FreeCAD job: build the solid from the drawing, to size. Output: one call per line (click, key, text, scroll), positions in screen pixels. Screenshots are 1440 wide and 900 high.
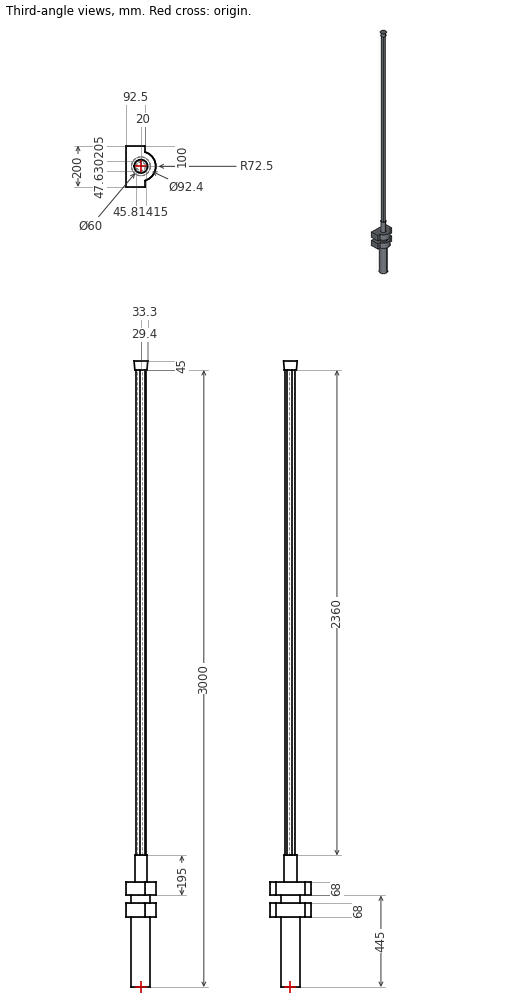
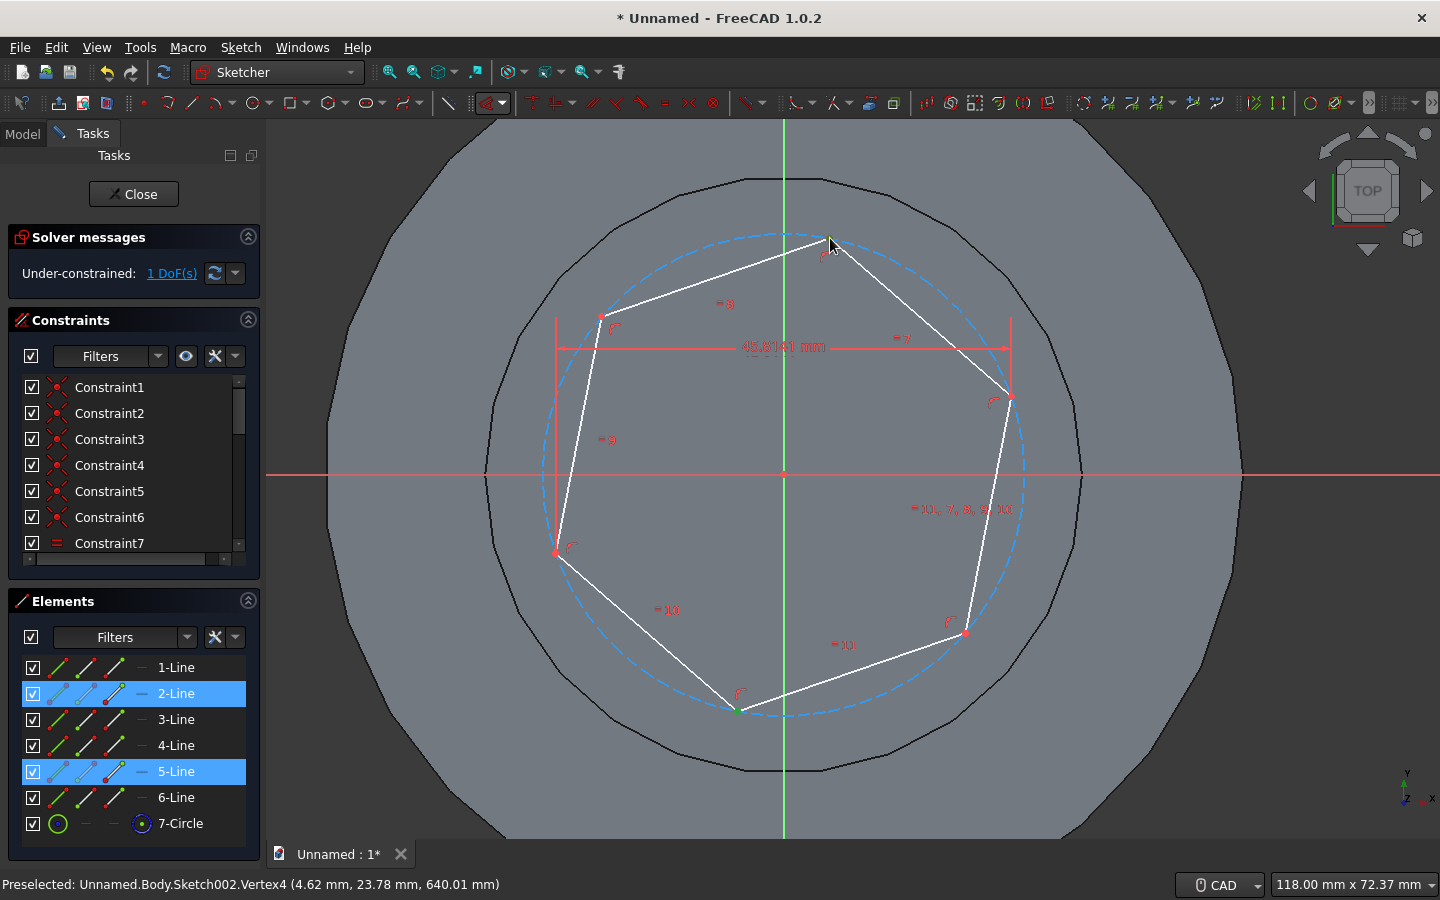
key(i)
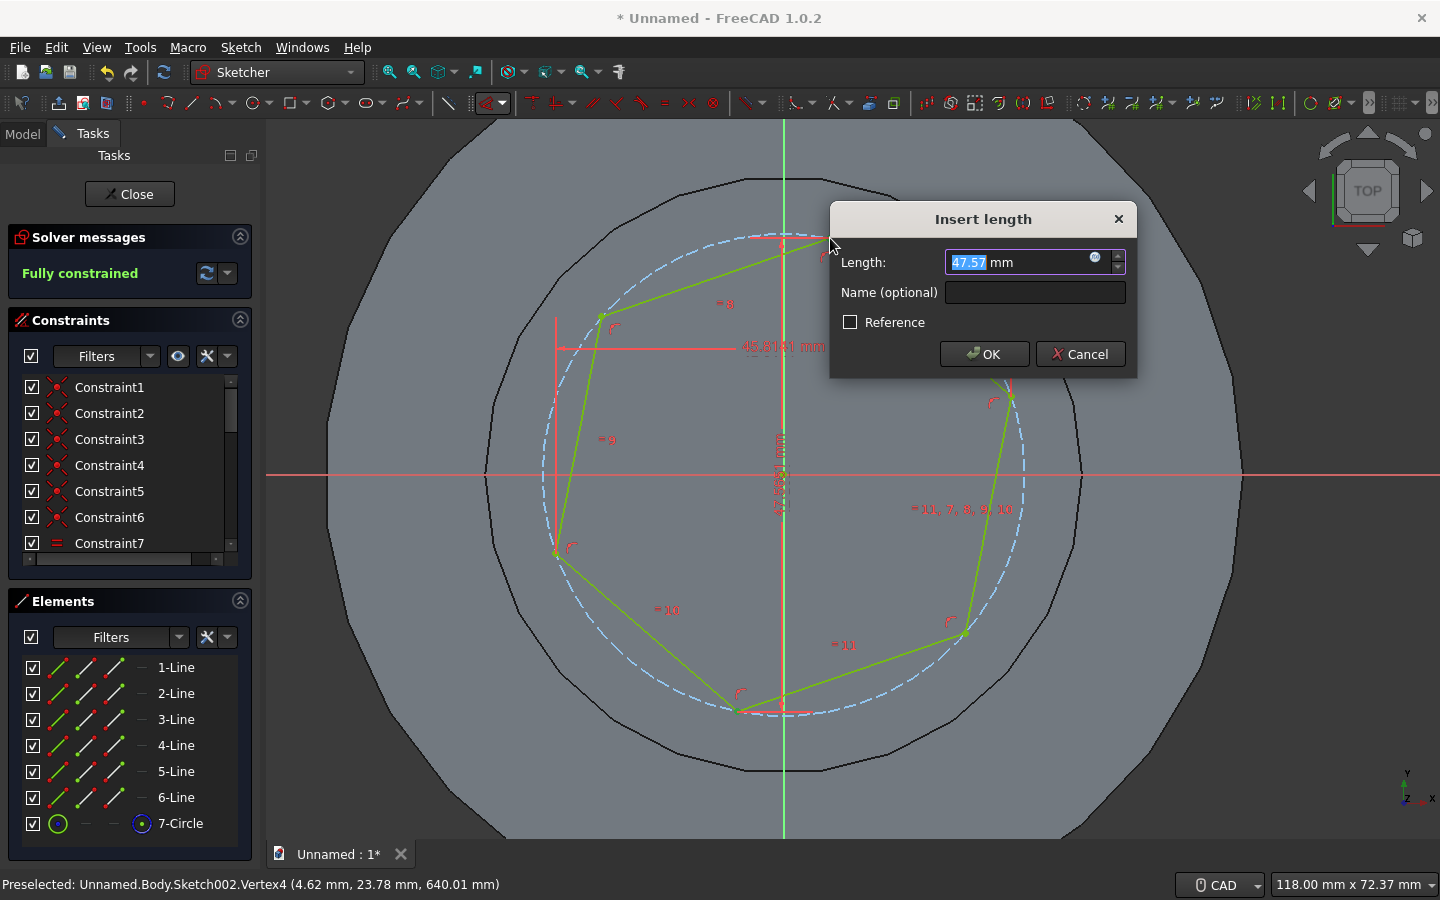
text(47.630205)
key(Return)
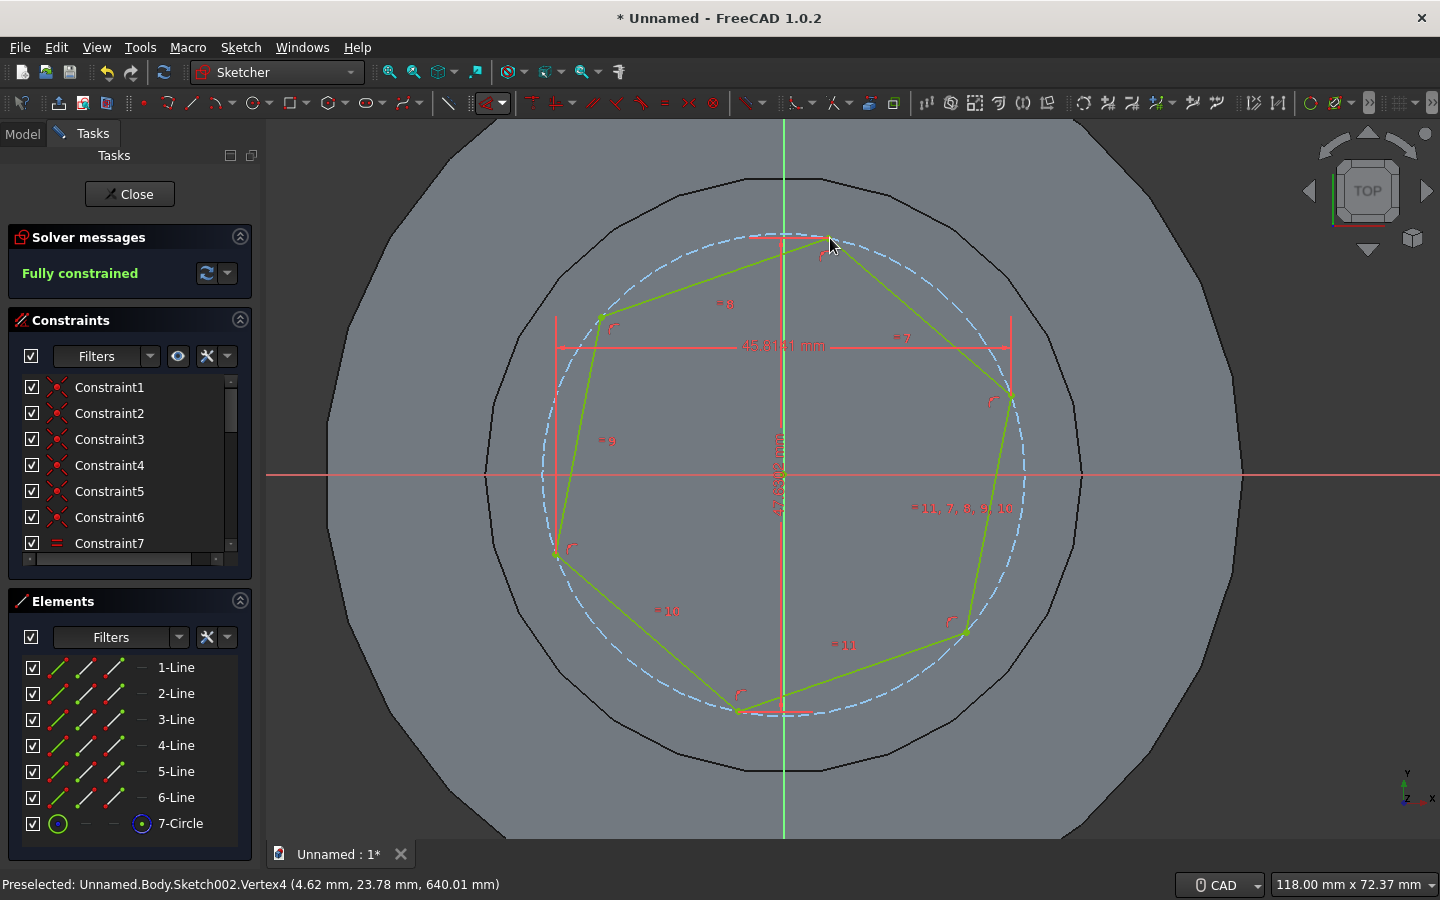
click(130, 194)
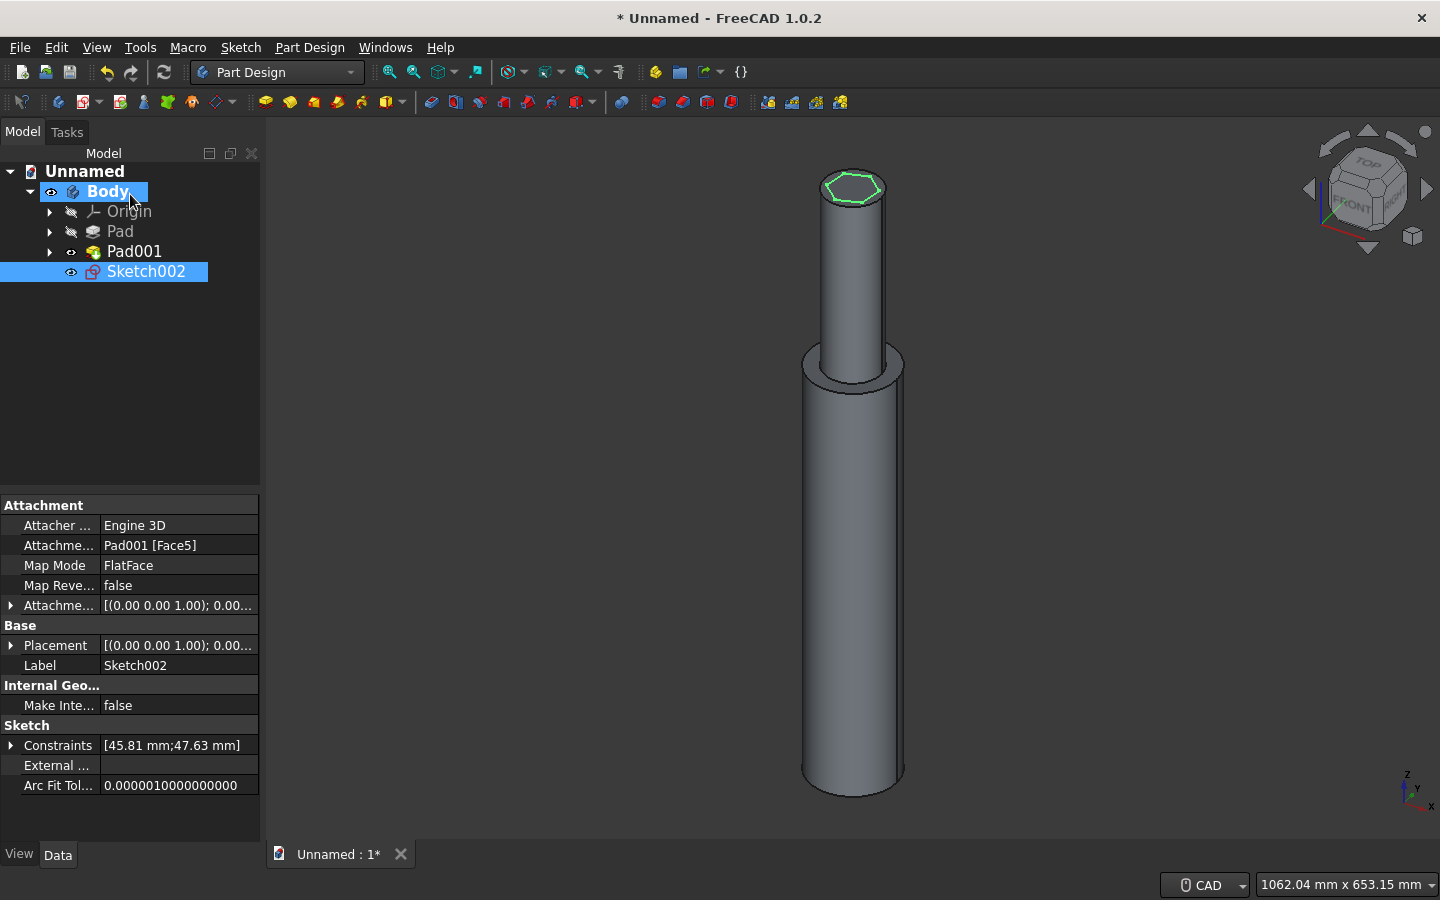
click(266, 102)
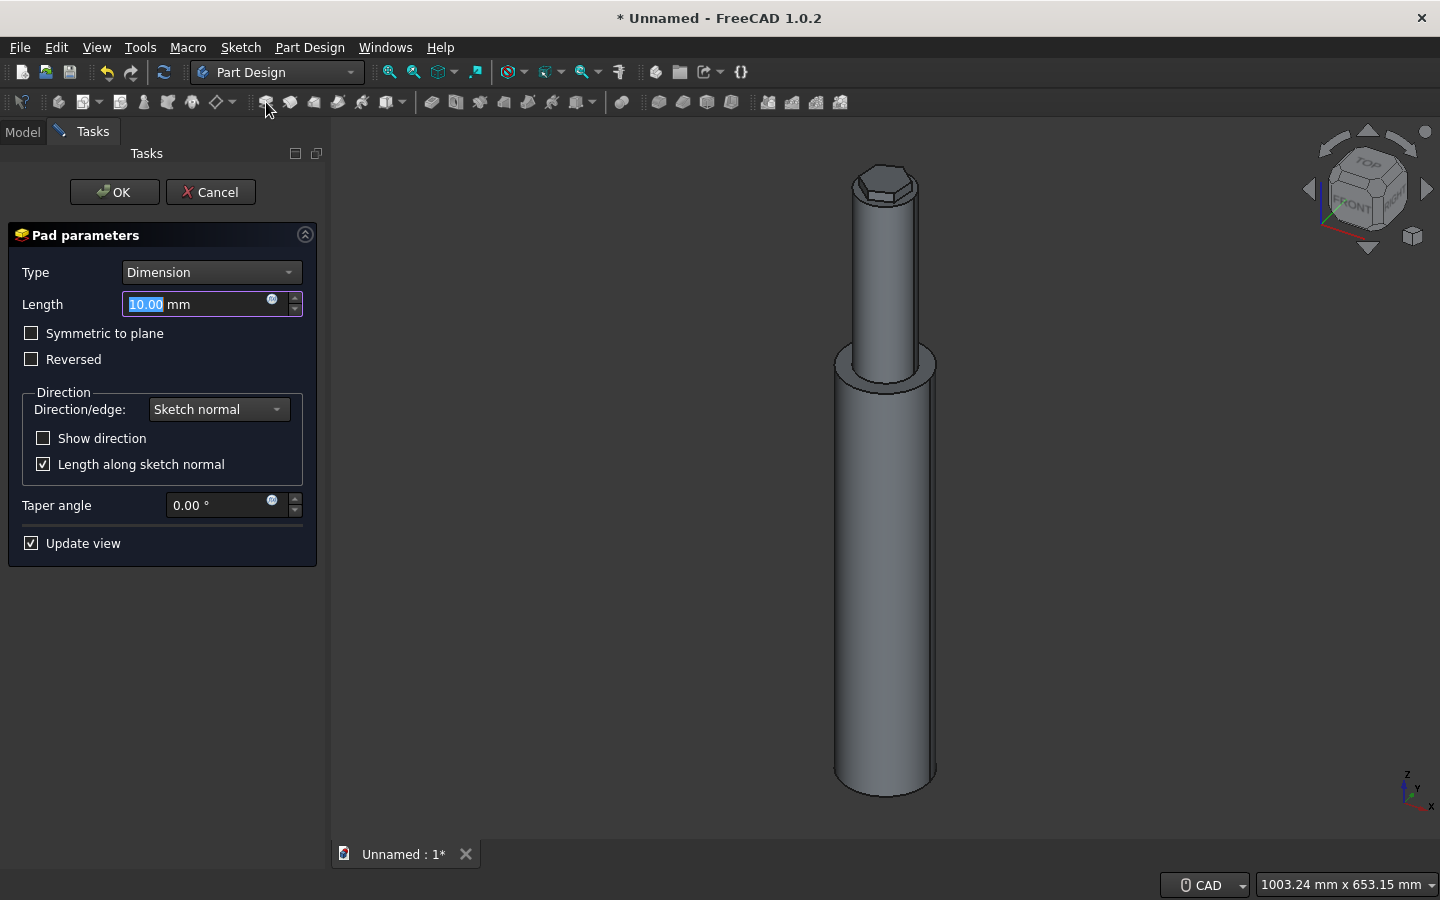
text(2360)
key(Tab)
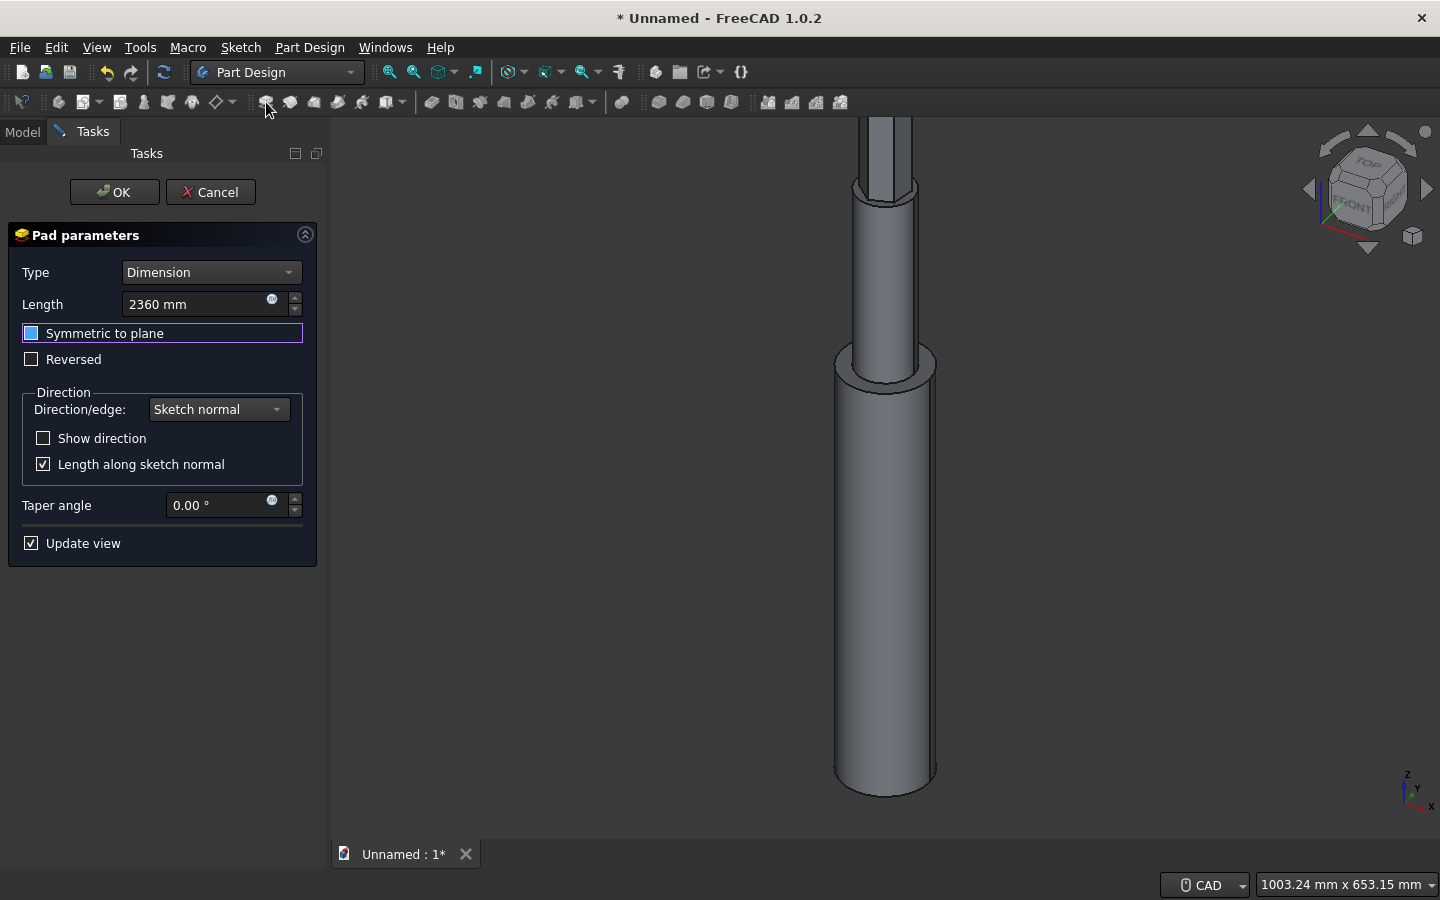
click(115, 192)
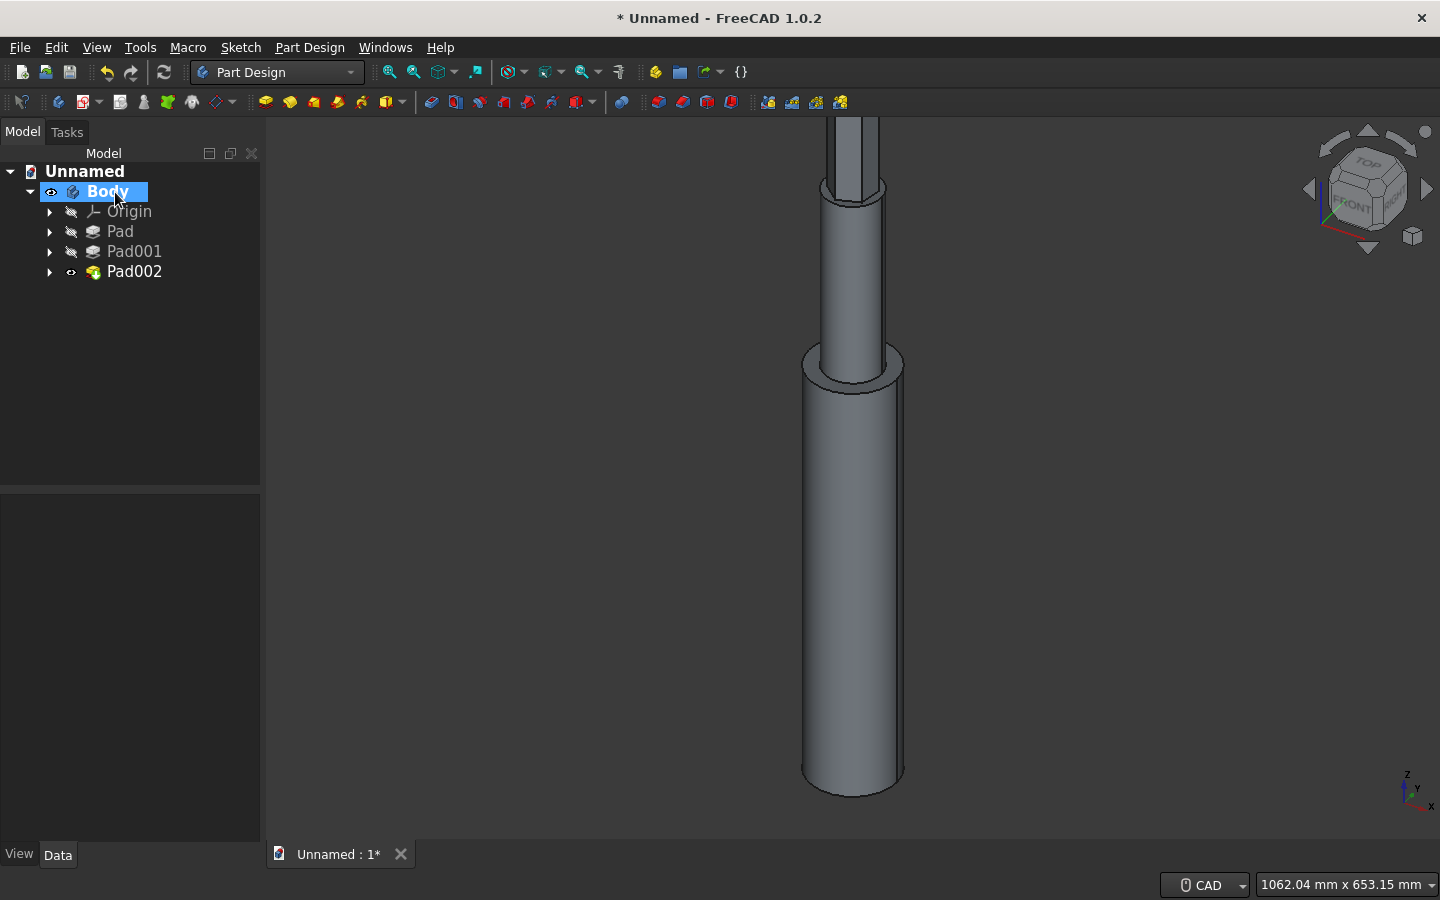
key(v)
key(f)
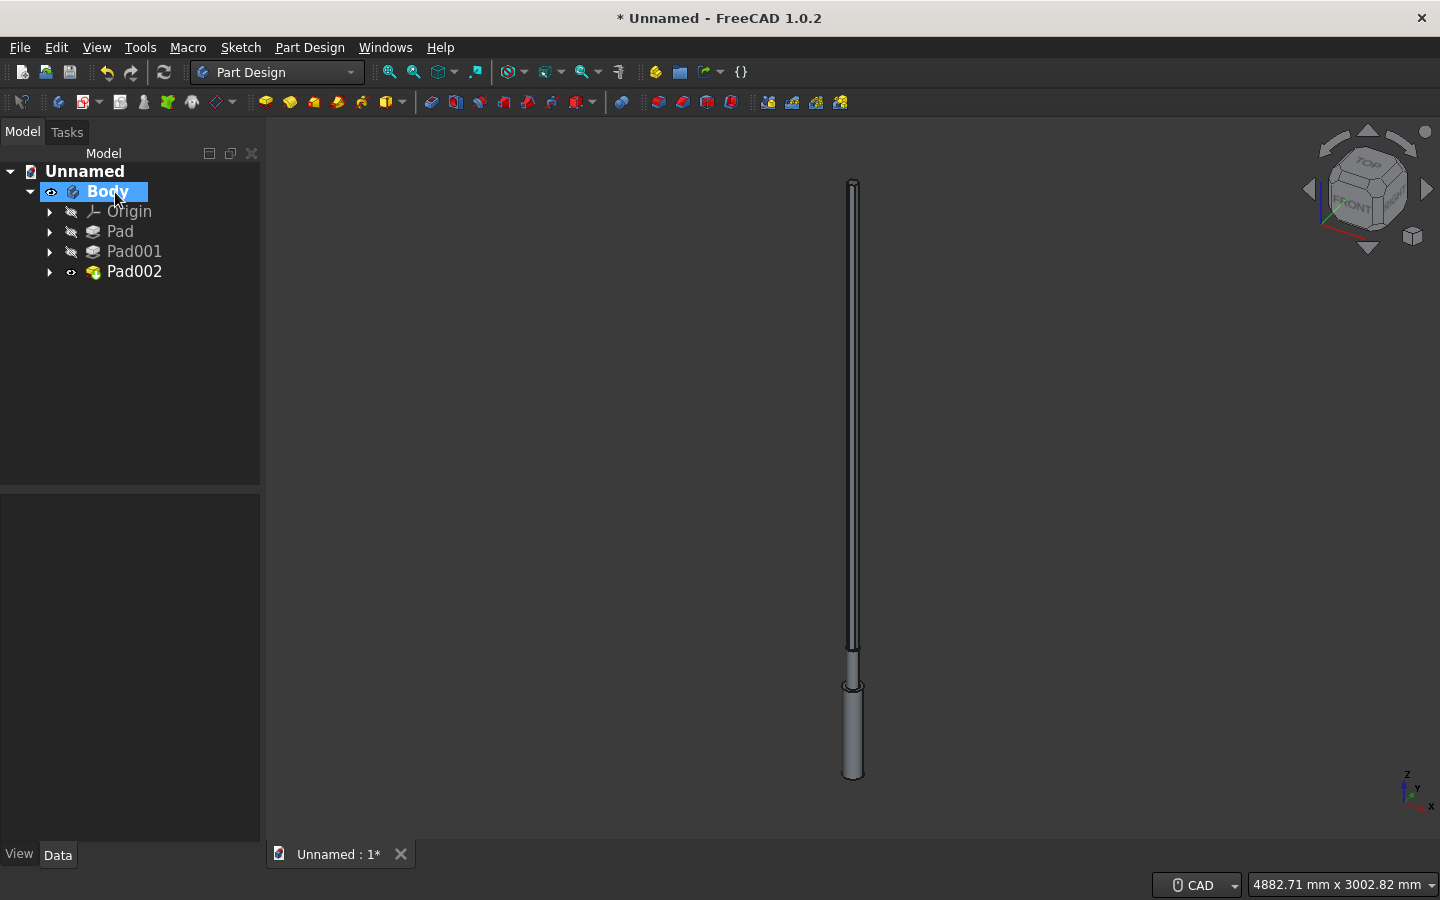
click(84, 102)